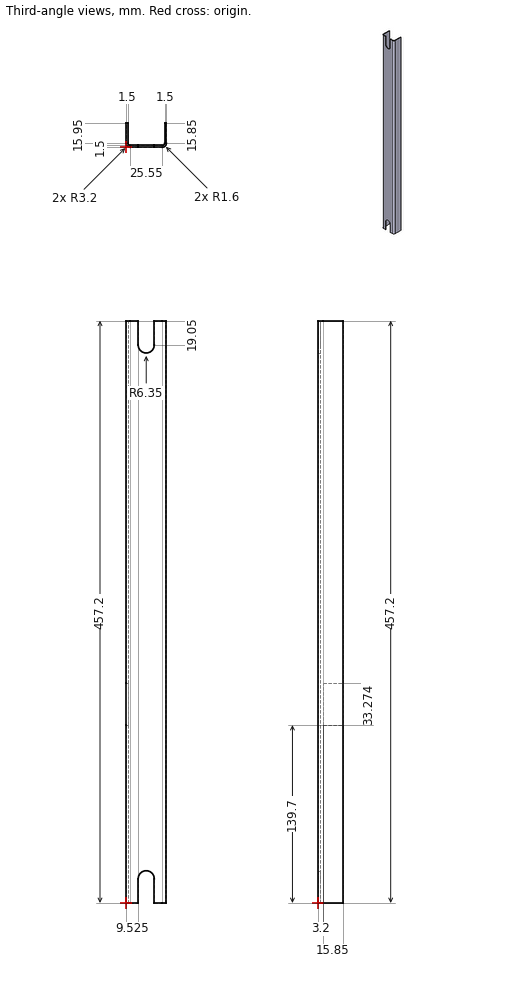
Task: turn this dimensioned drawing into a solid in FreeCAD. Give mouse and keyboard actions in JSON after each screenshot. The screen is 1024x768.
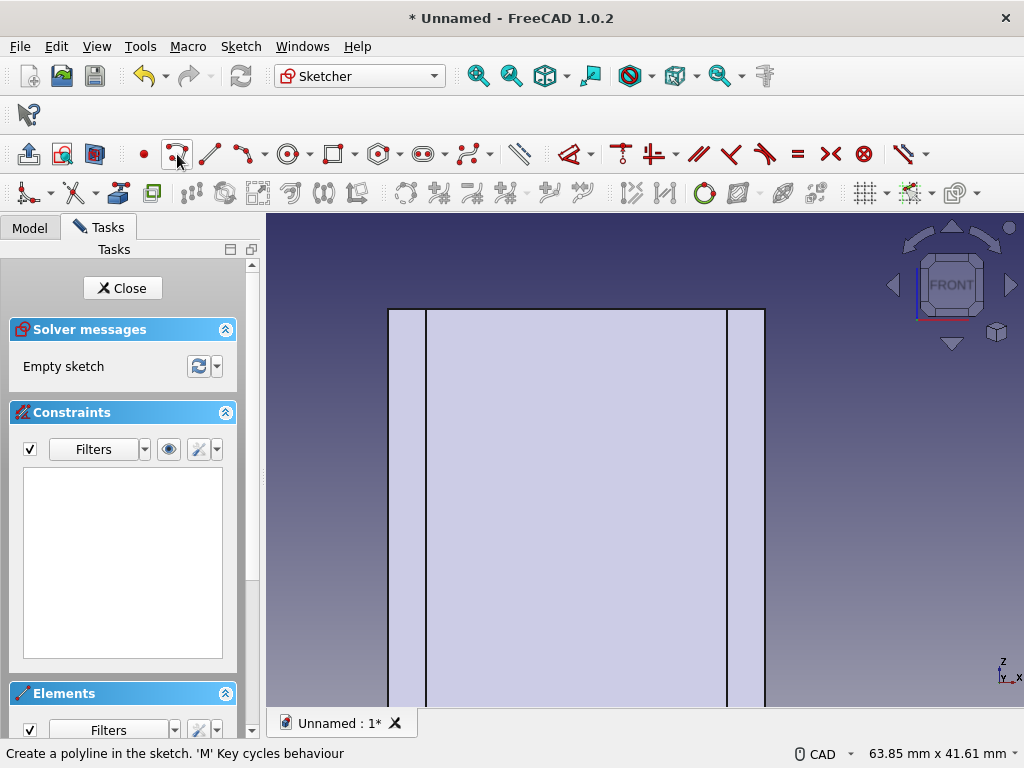
{"action": "left_click", "coordinate": [652, 535]}
{"action": "left_click", "coordinate": [652, 309]}
{"action": "left_click", "coordinate": [501, 309]}
{"action": "left_click", "coordinate": [501, 535]}
{"action": "right_click", "coordinate": [501, 535]}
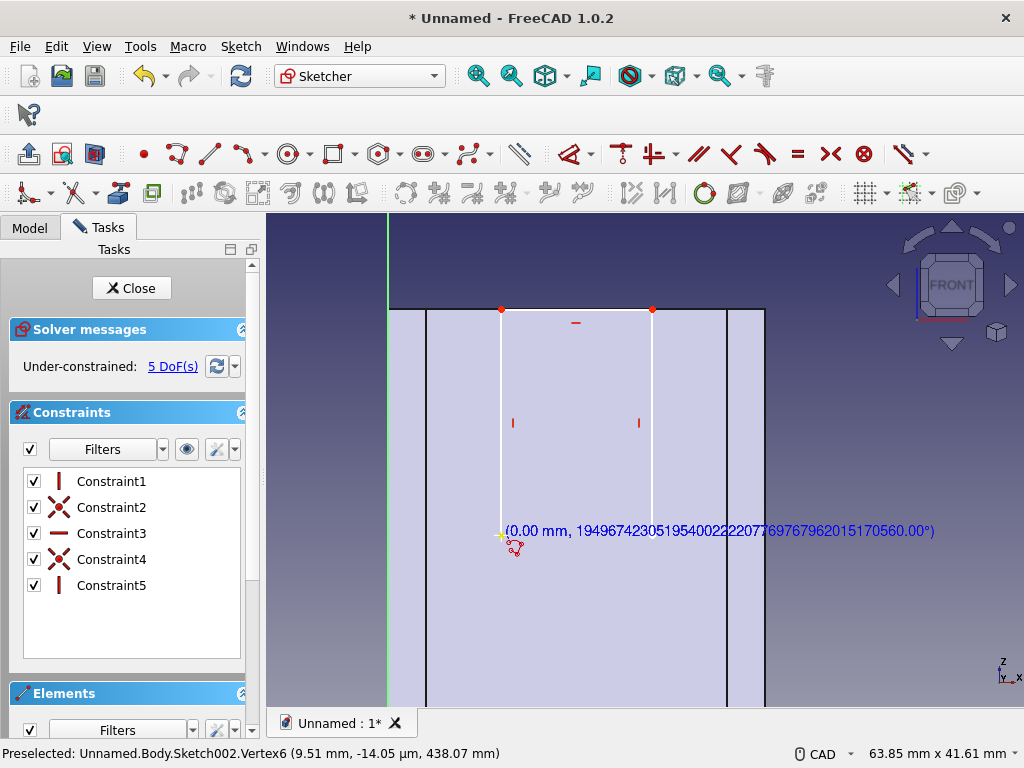
{"action": "key", "text": "g 3 a"}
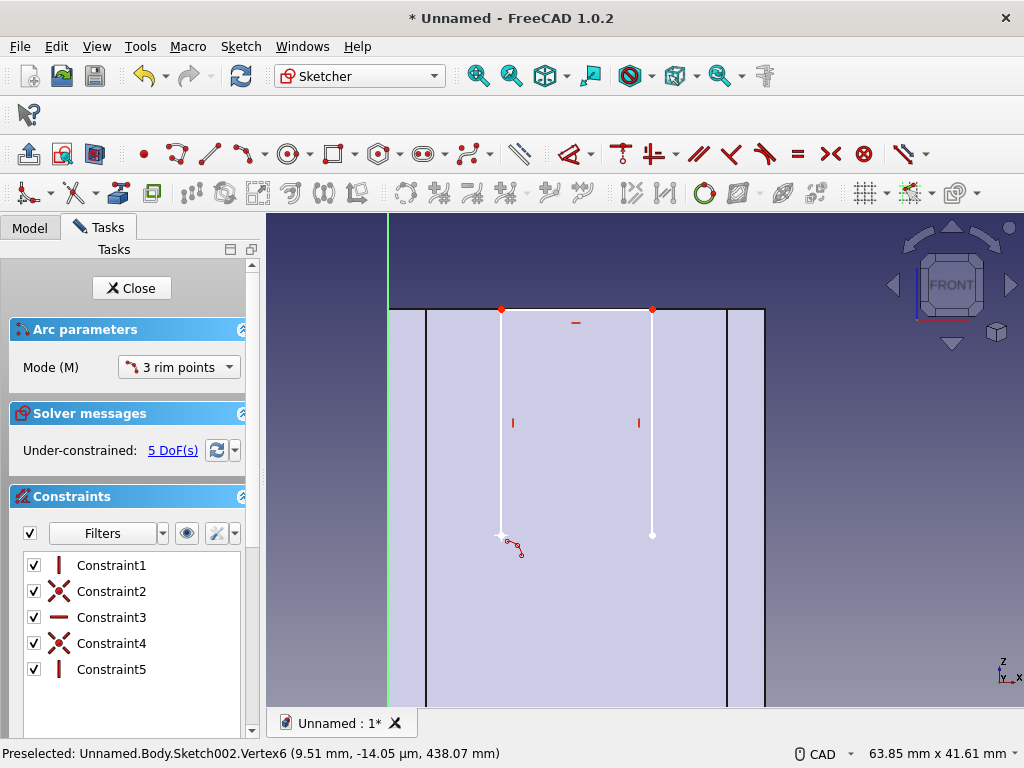
{"action": "left_click", "coordinate": [501, 536]}
{"action": "left_click", "coordinate": [652, 536]}
{"action": "left_click", "coordinate": [577, 610]}
{"action": "key", "text": "Escape"}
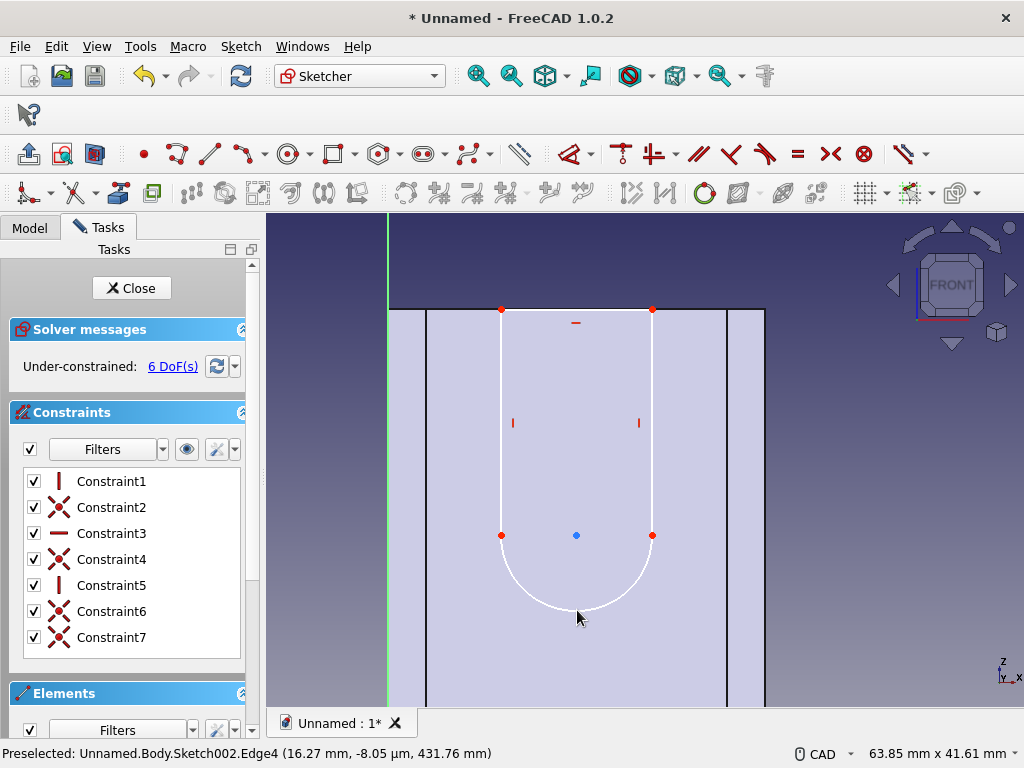
{"action": "left_click", "coordinate": [652, 468]}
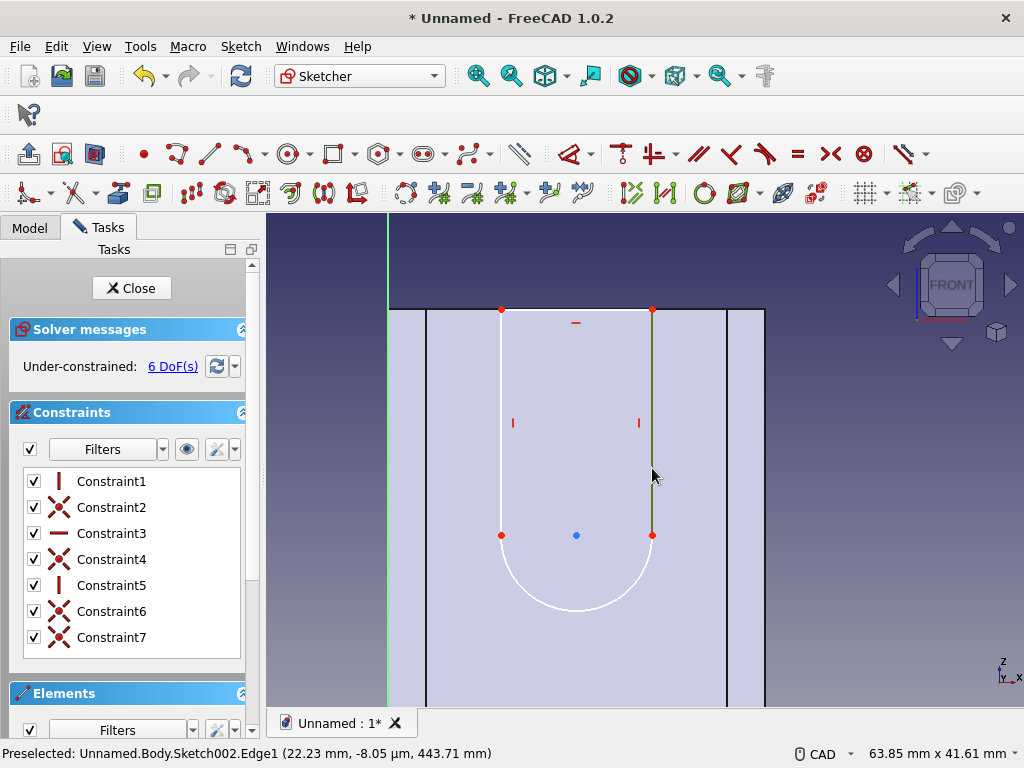
{"action": "left_click", "coordinate": [532, 597]}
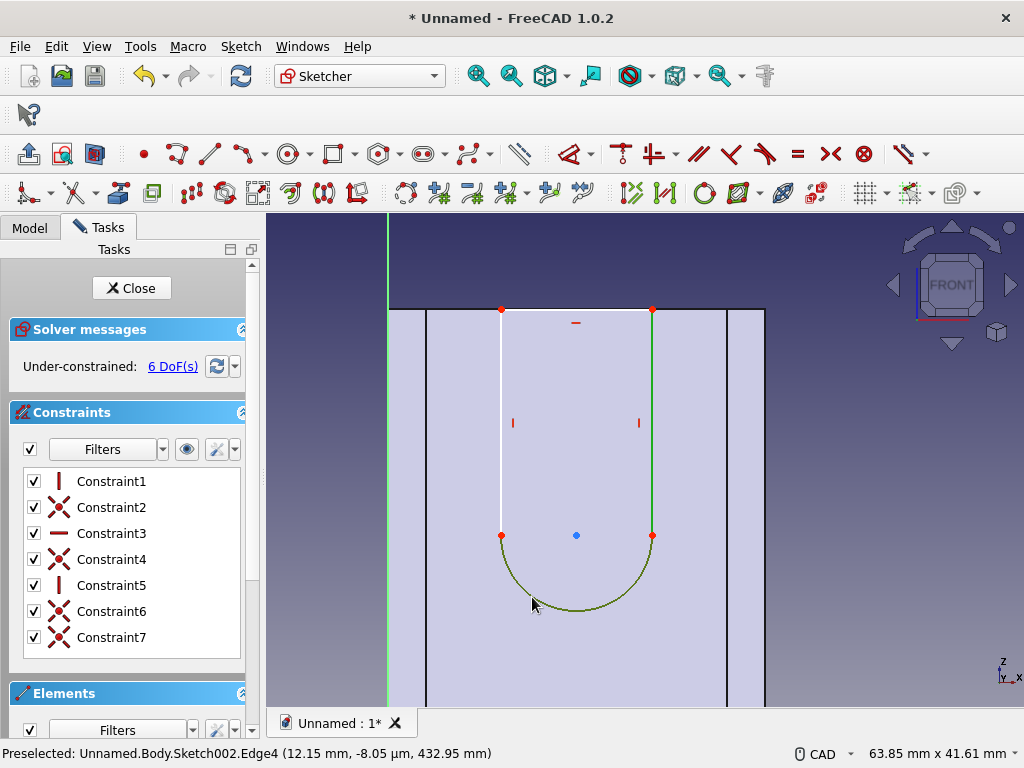
{"action": "left_click", "coordinate": [765, 154]}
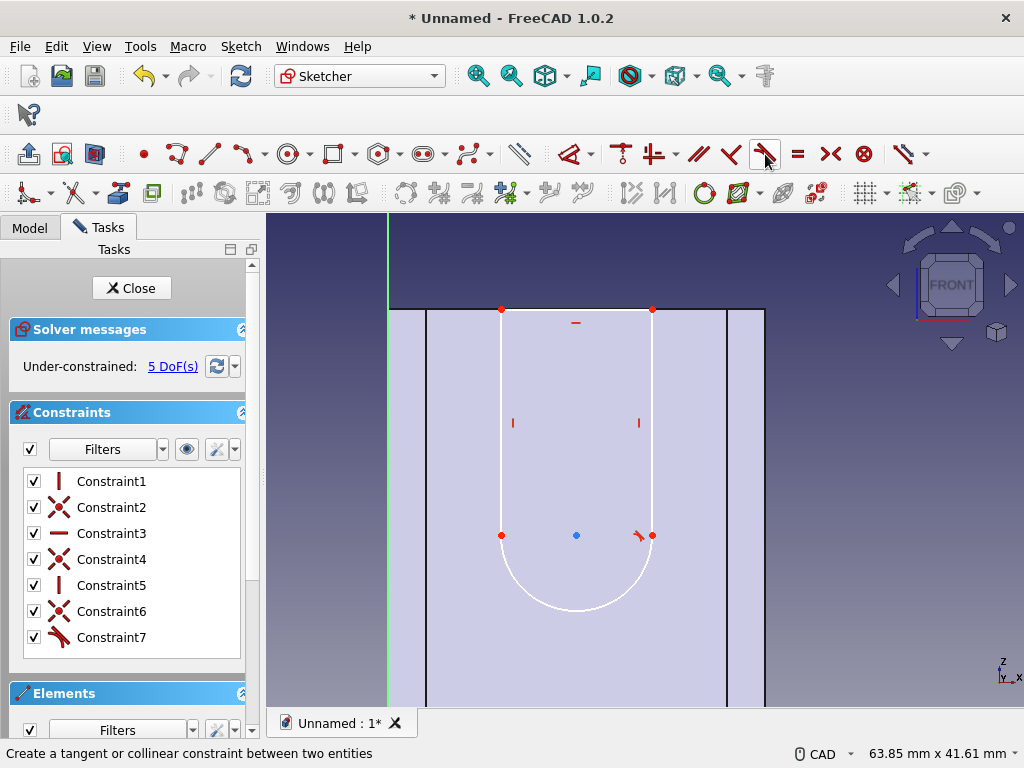
{"action": "left_click", "coordinate": [501, 378]}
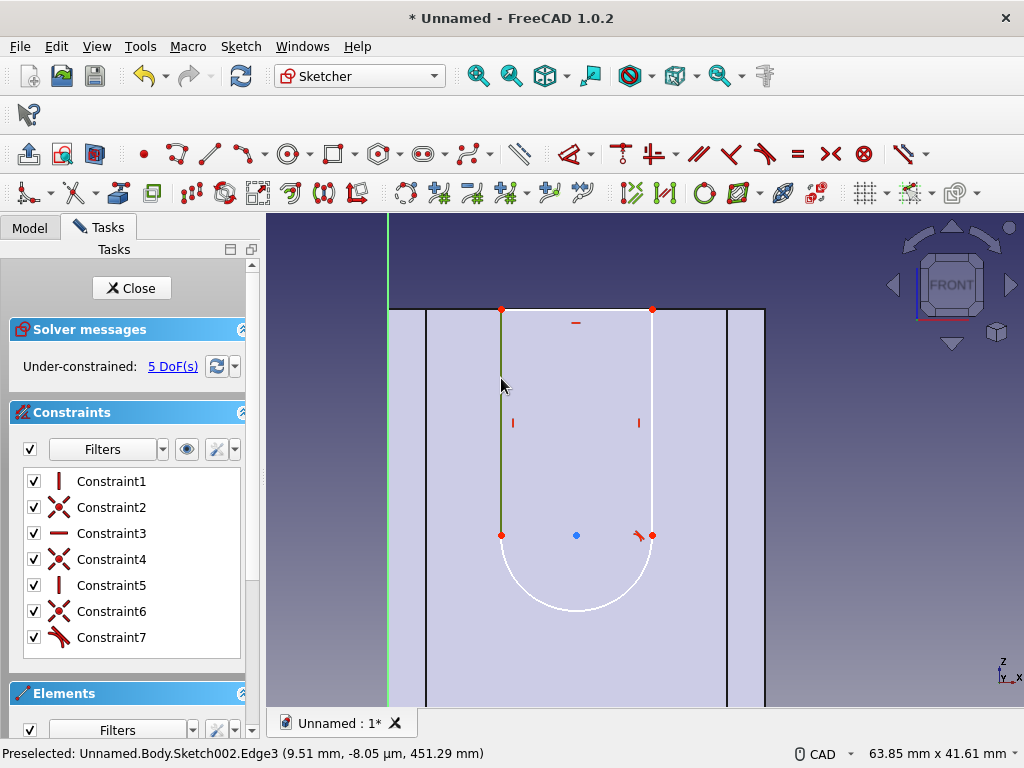
{"action": "left_click", "coordinate": [532, 597]}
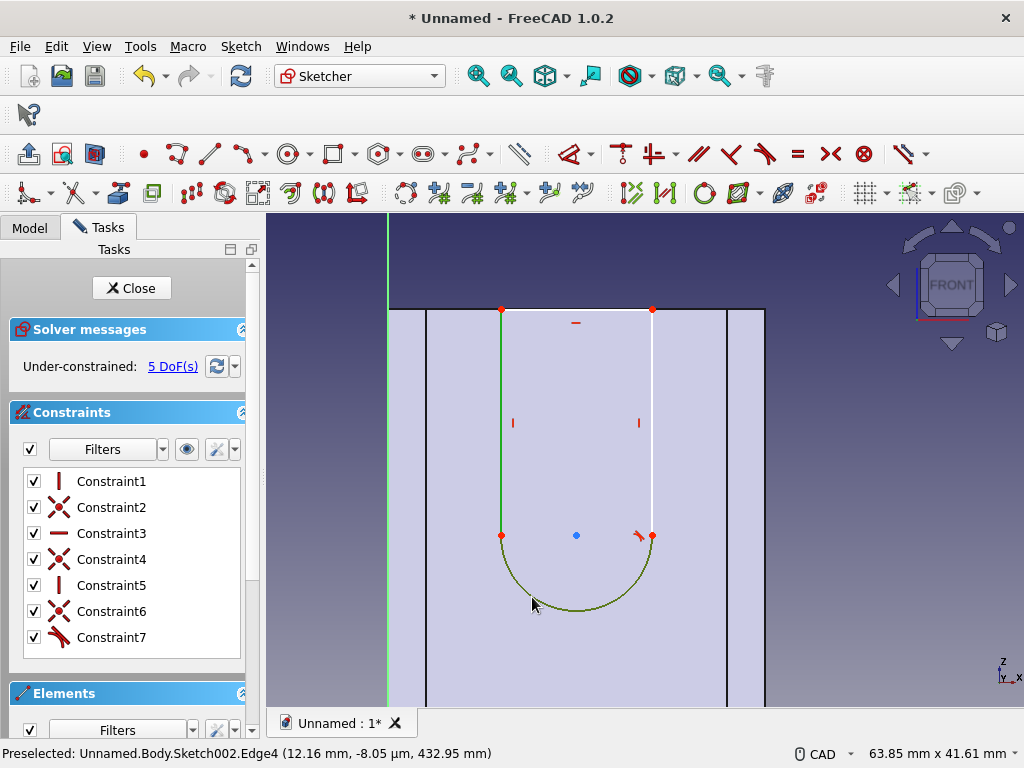
{"action": "key", "text": "t"}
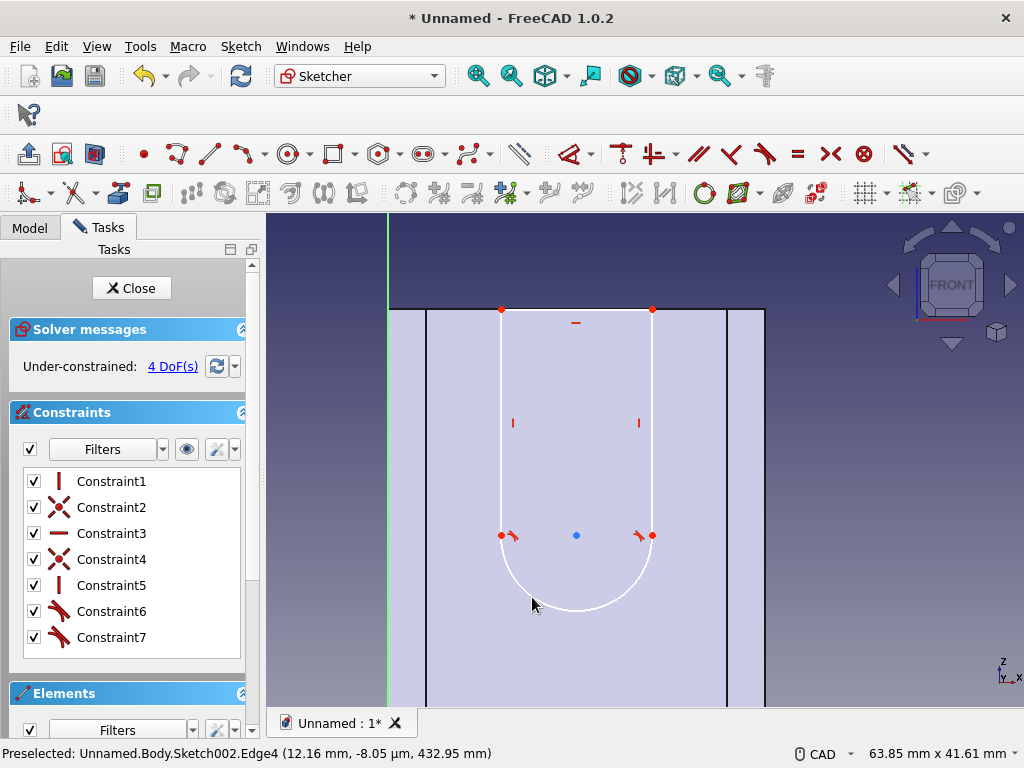
{"action": "key", "text": "d"}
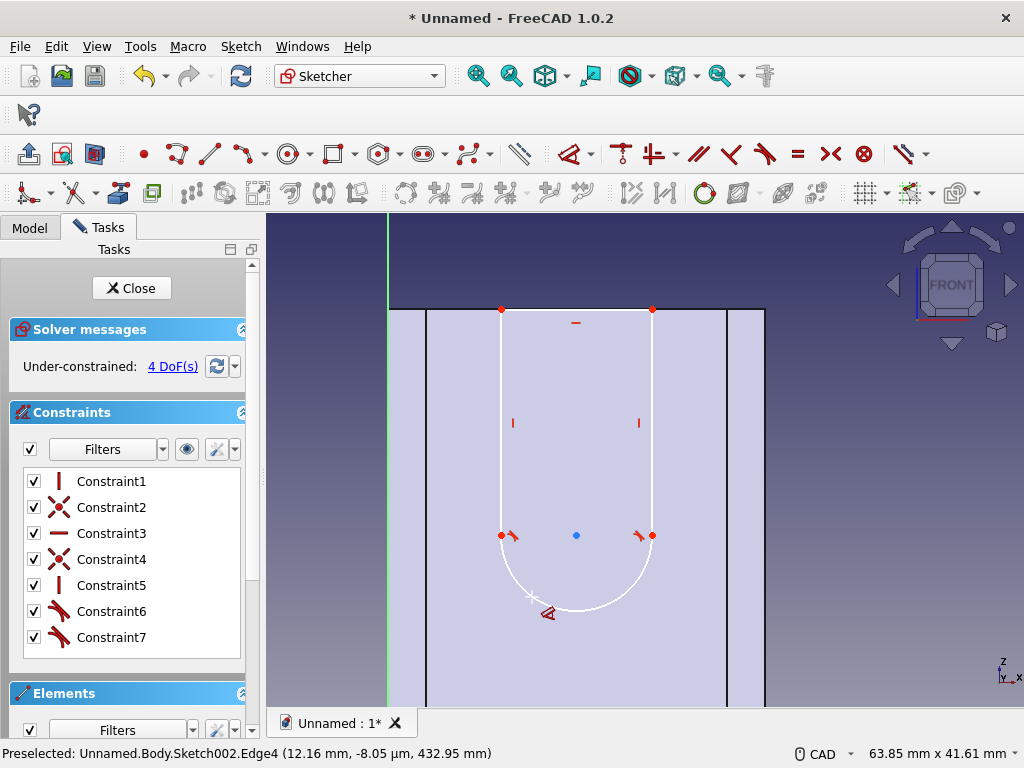
{"action": "left_click", "coordinate": [532, 597]}
{"action": "left_click", "coordinate": [513, 623]}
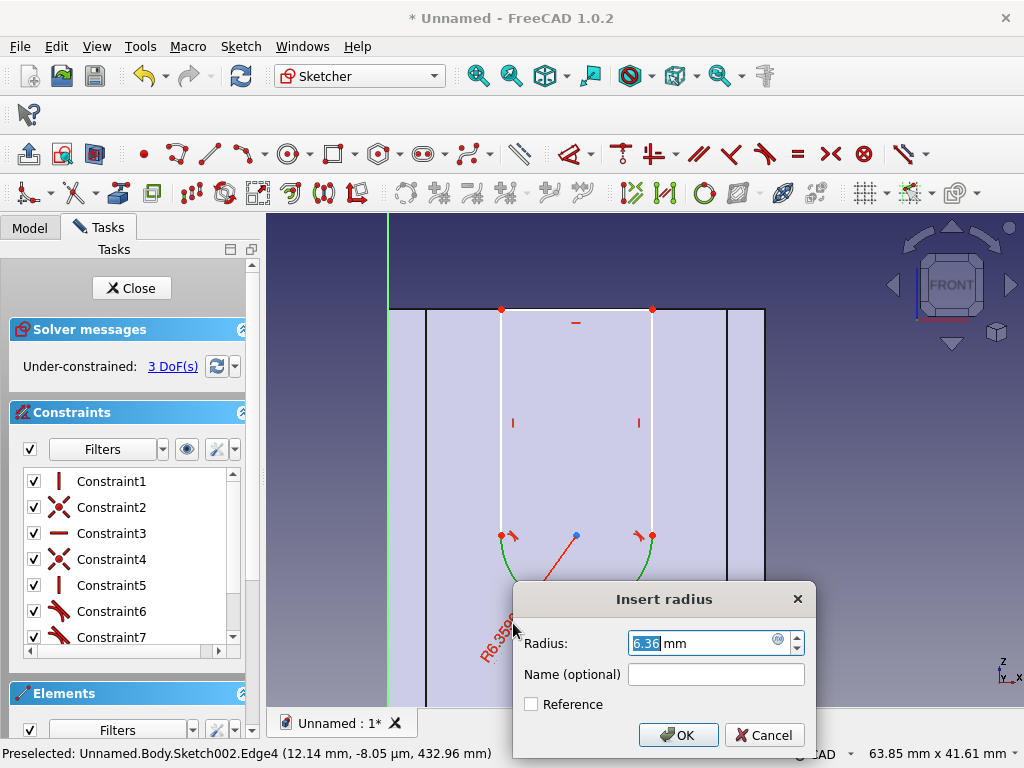
{"action": "type", "text": "6.35"}
{"action": "key", "text": "Return"}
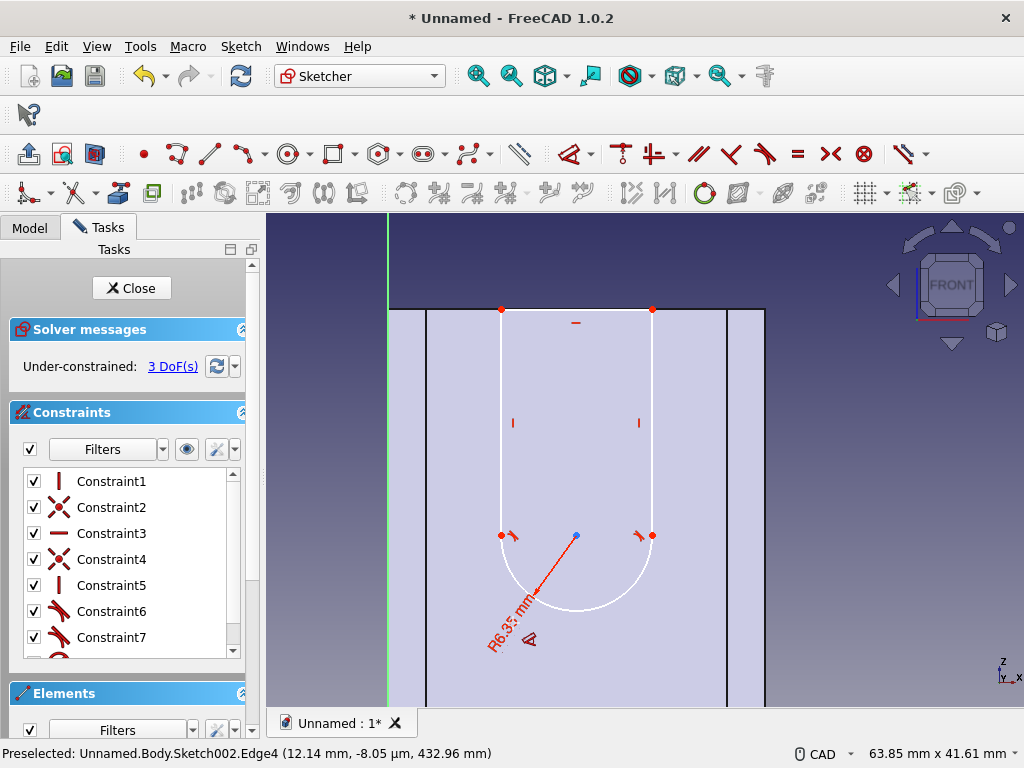
{"action": "left_click", "coordinate": [652, 468]}
{"action": "left_click", "coordinate": [686, 423]}